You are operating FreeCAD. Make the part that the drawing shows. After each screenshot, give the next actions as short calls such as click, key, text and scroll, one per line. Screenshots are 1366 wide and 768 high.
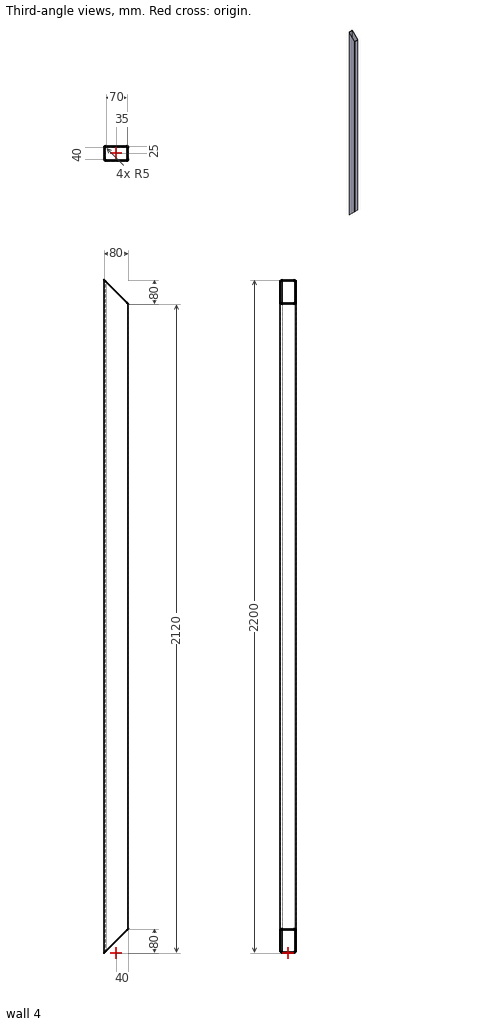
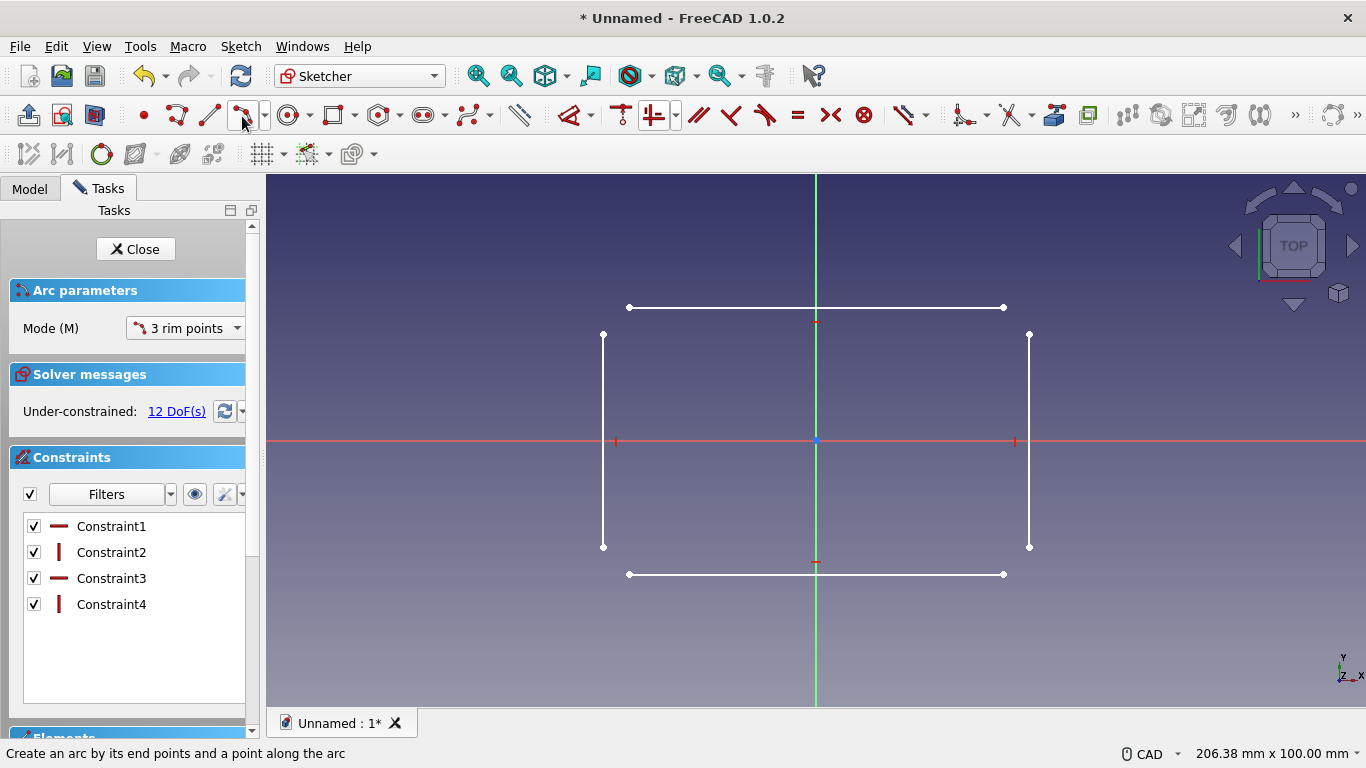
click(629, 308)
click(603, 335)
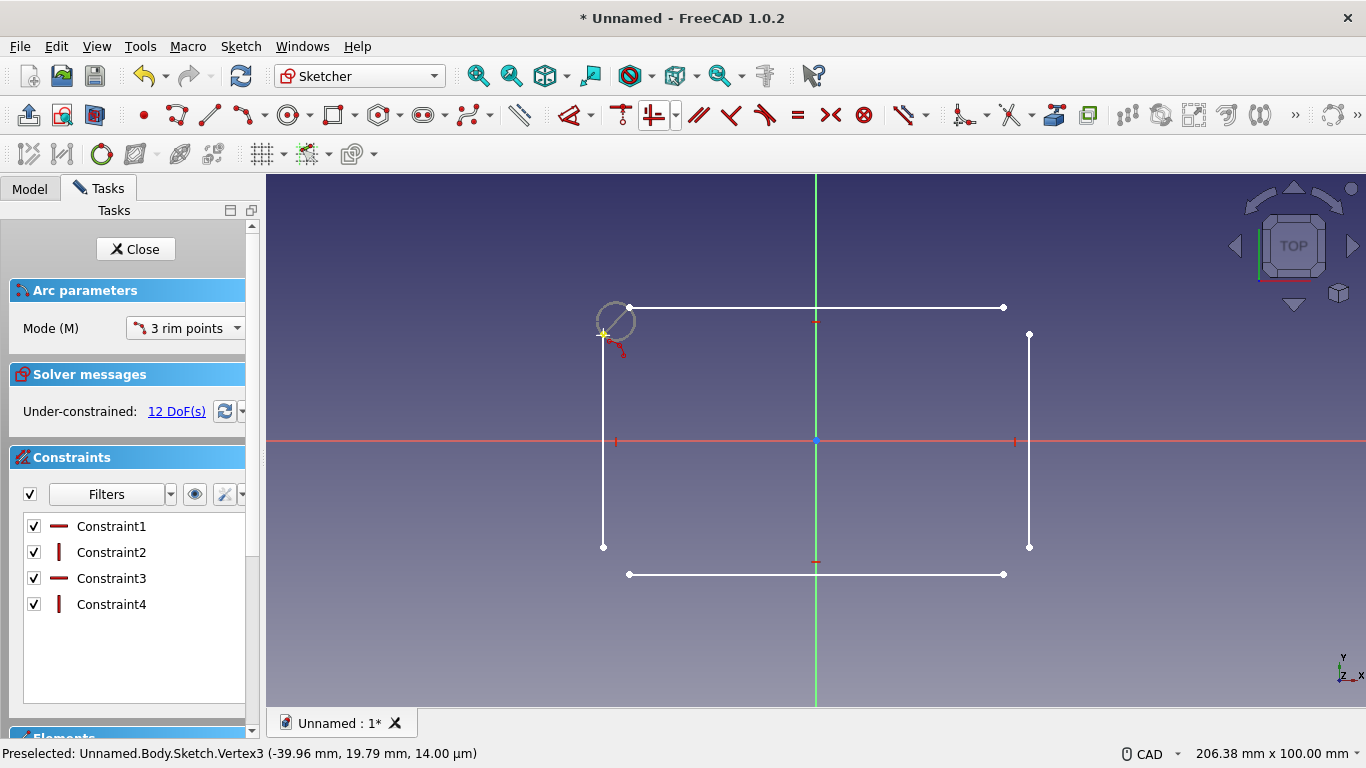
scroll(611, 315, up, 4)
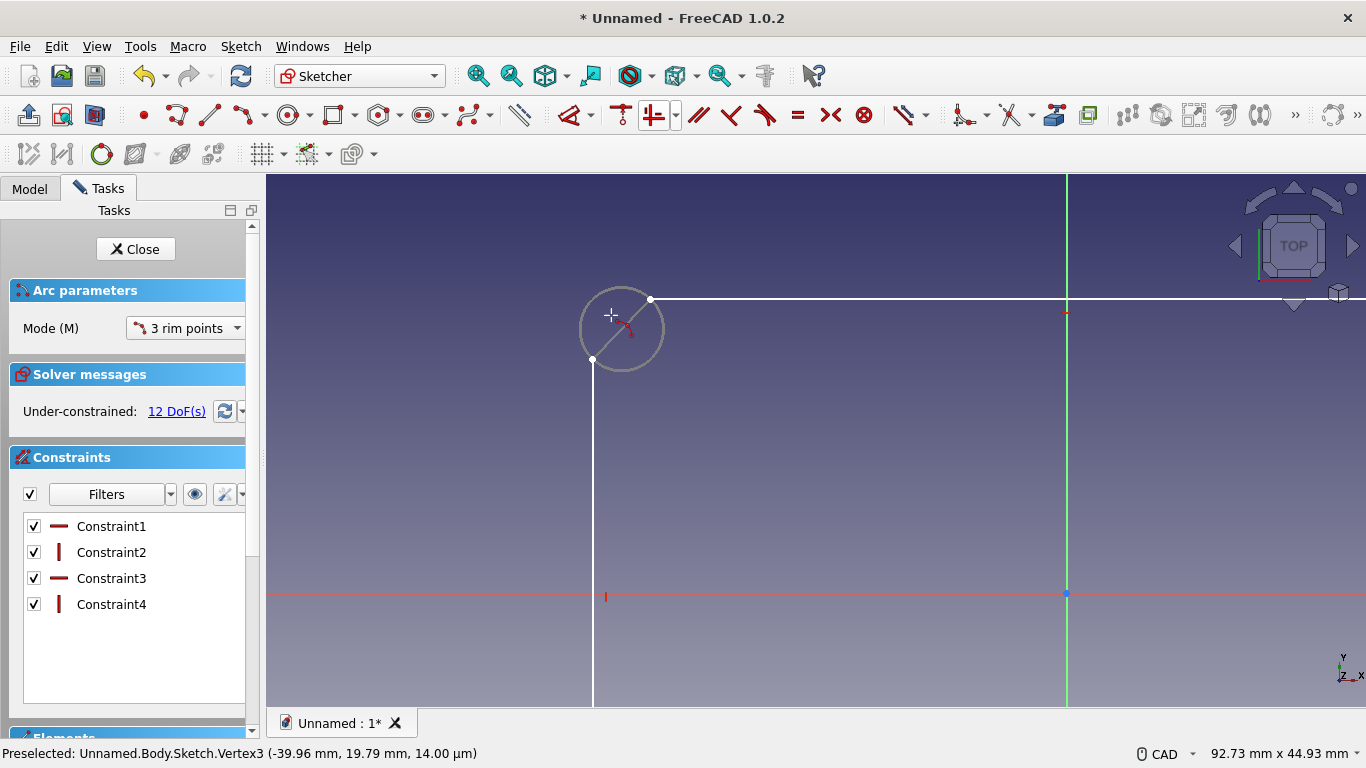
click(610, 315)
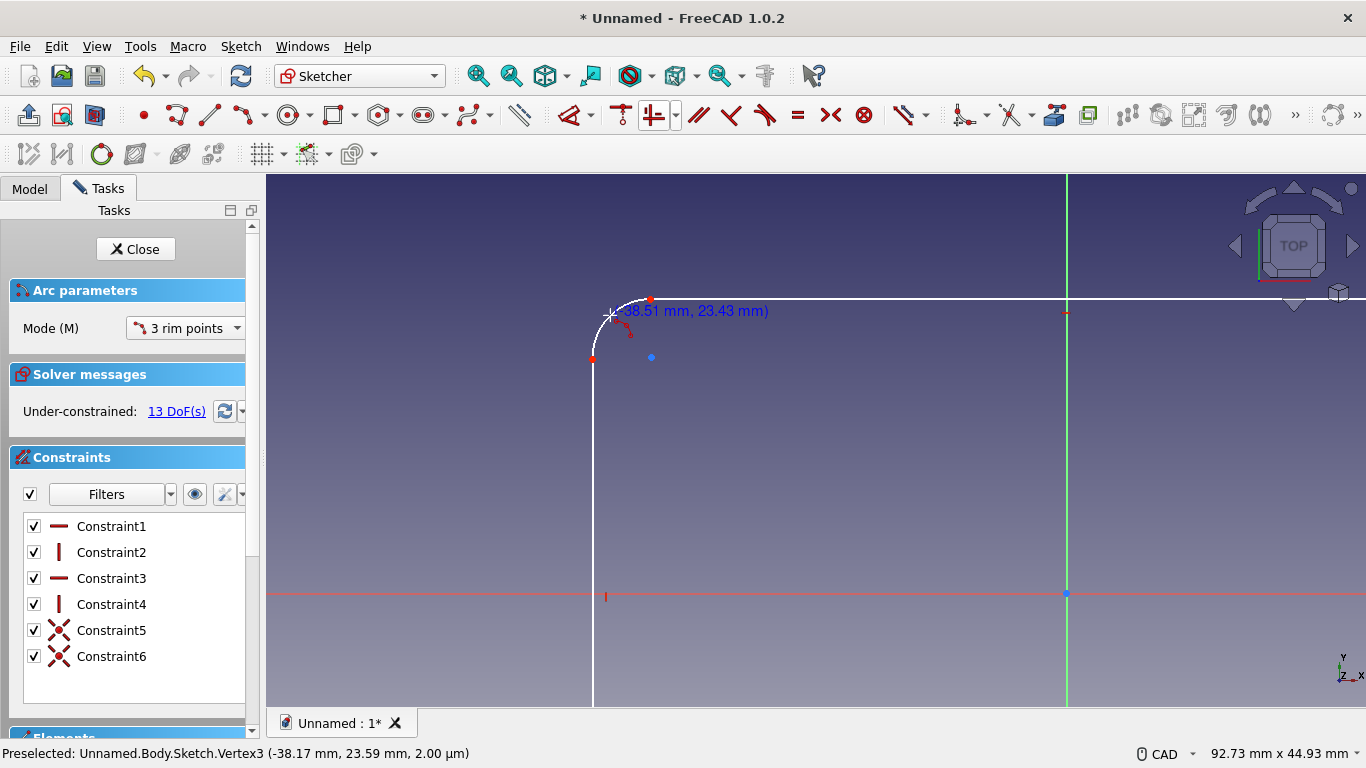
scroll(359, 254, down, 3)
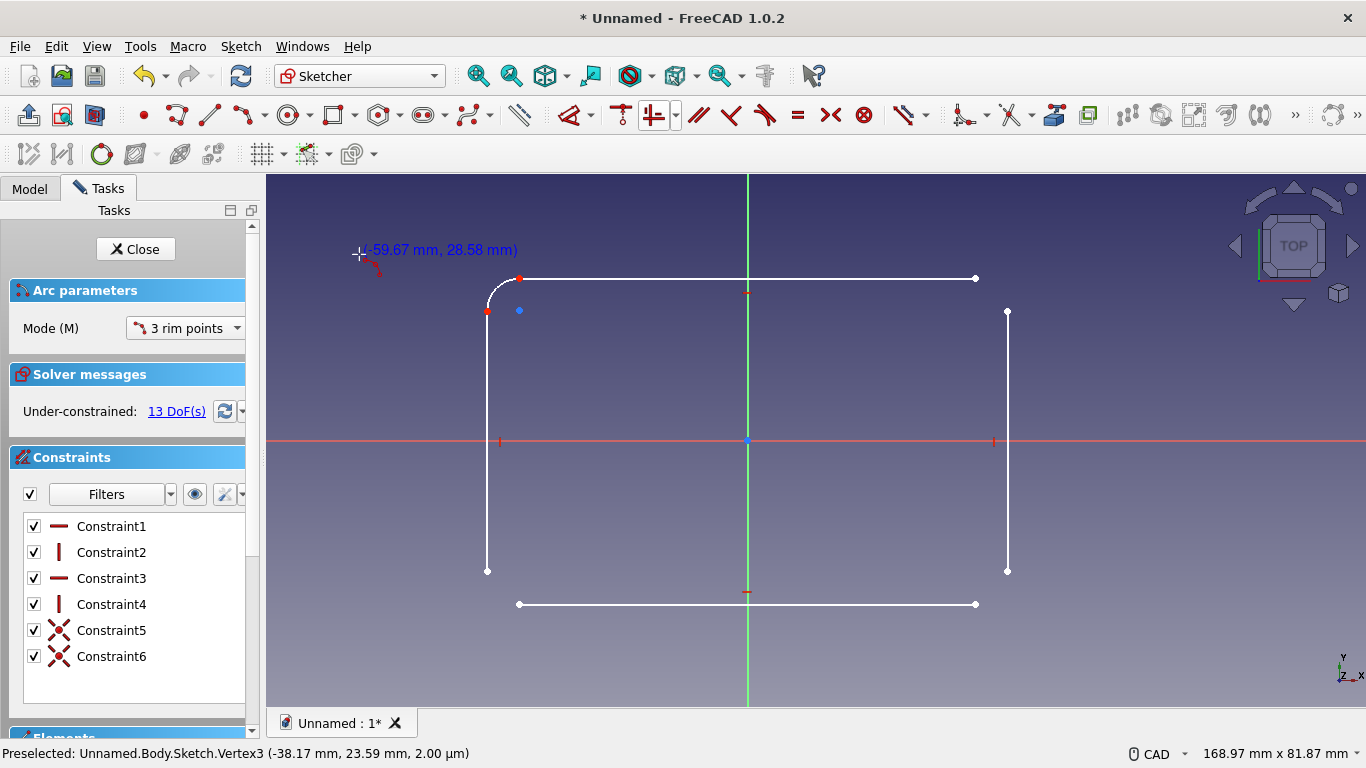
click(487, 572)
click(519, 605)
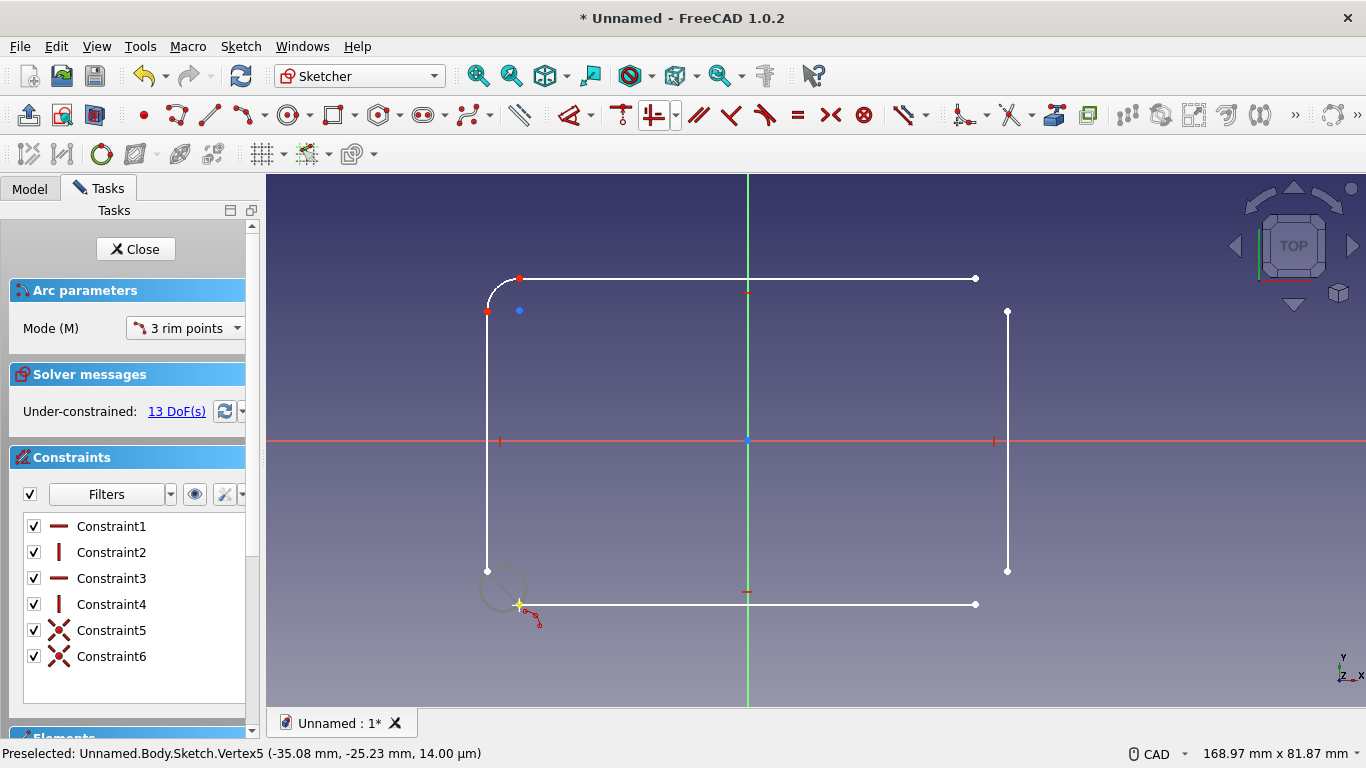
scroll(497, 594, up, 3)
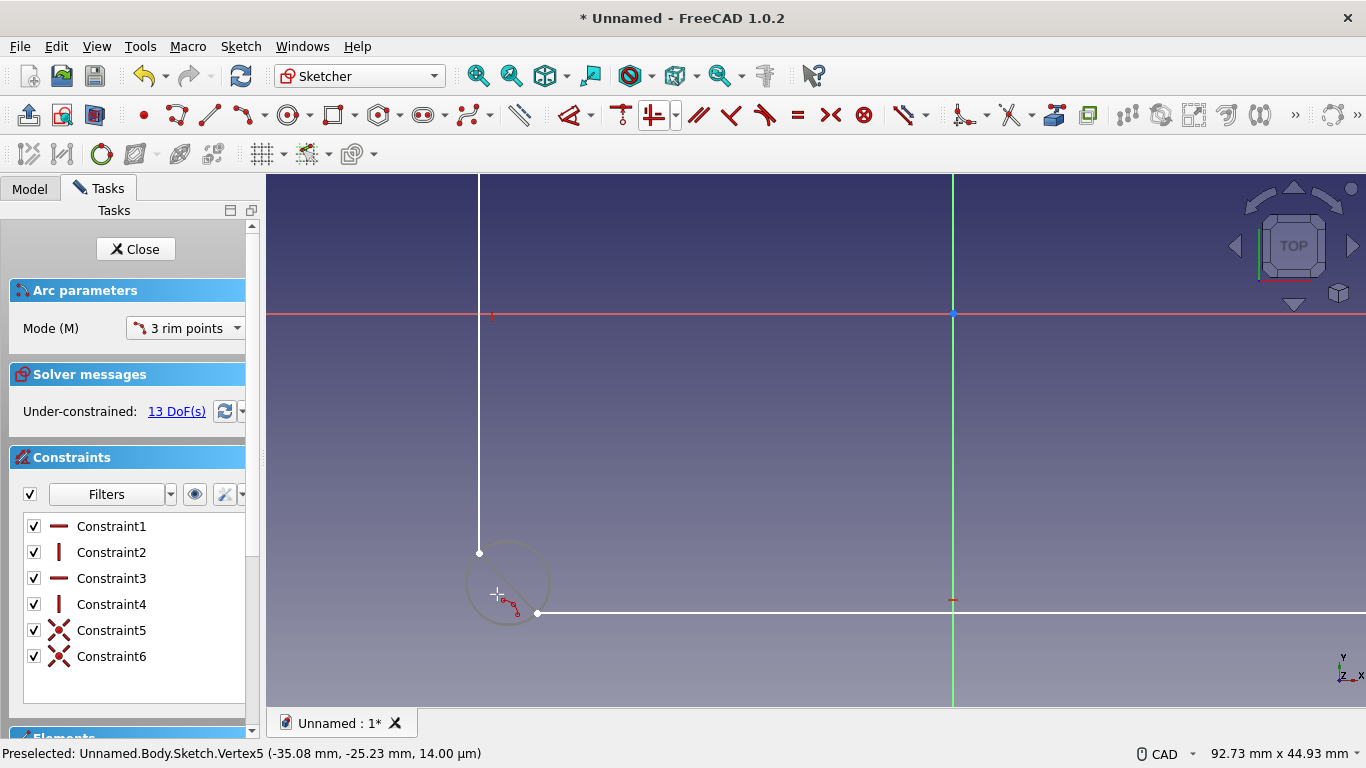
click(496, 593)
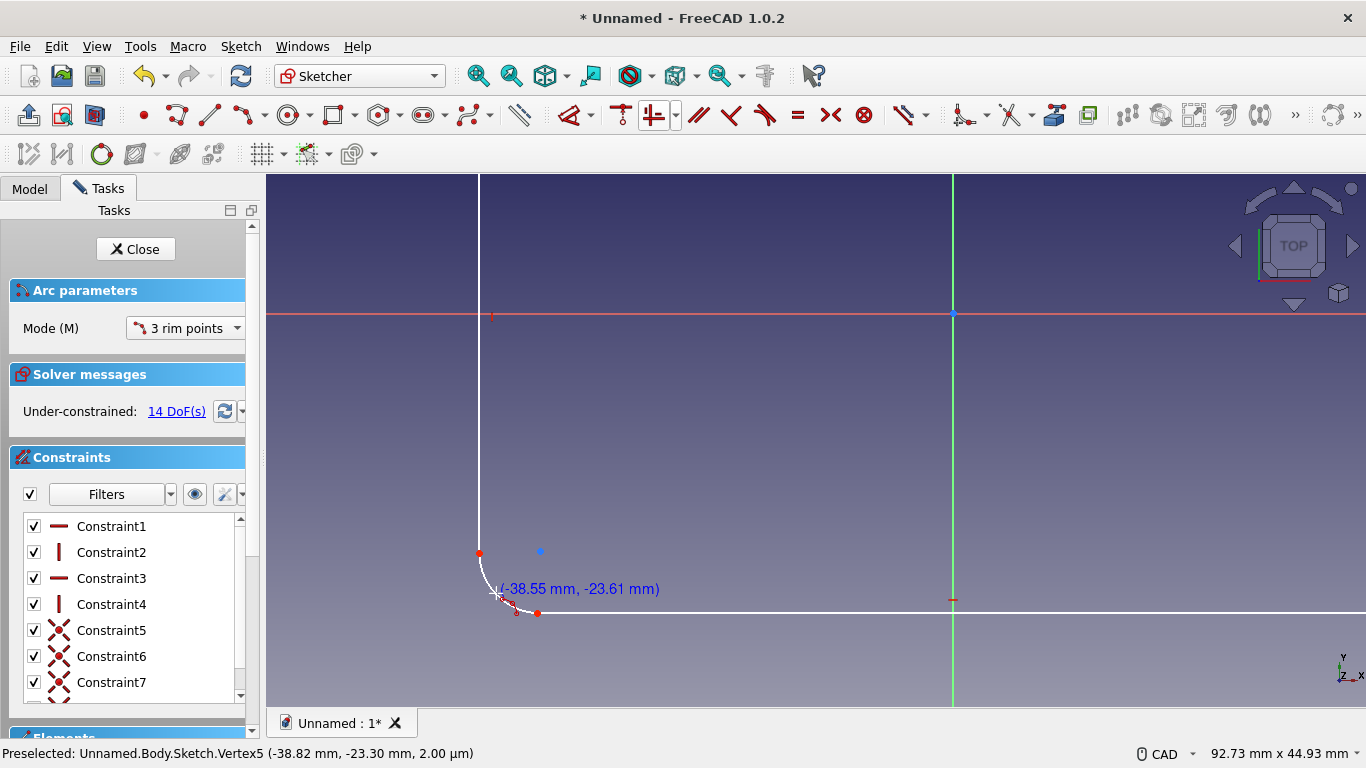
scroll(497, 594, down, 3)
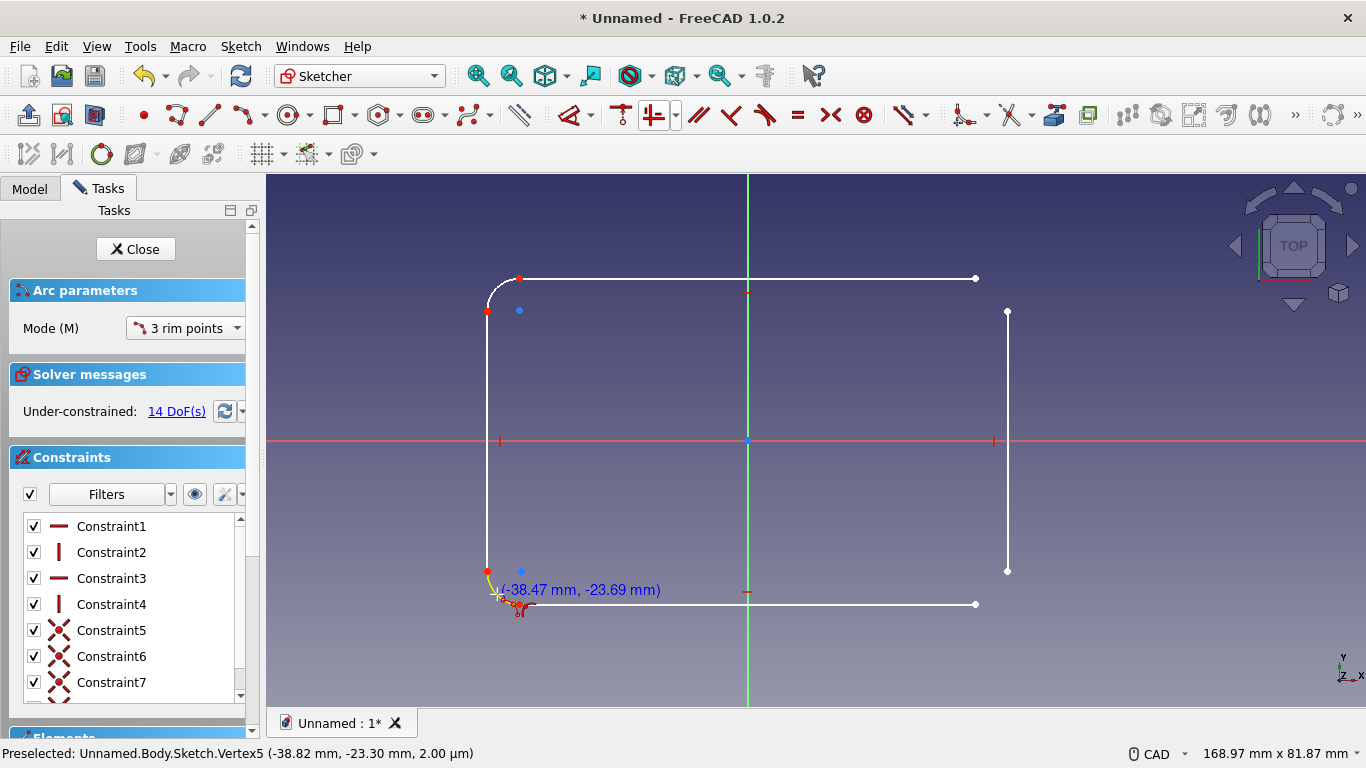
click(976, 605)
click(1008, 572)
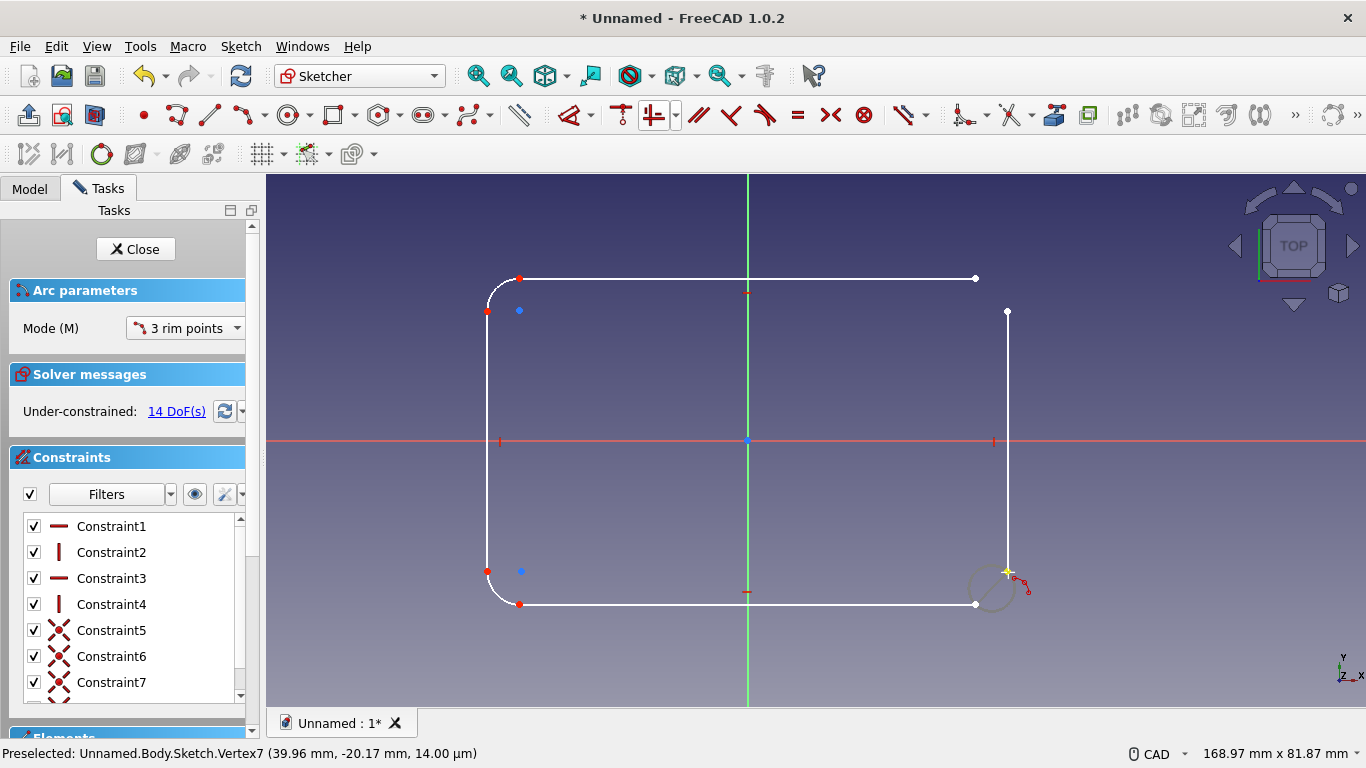
scroll(998, 594, up, 3)